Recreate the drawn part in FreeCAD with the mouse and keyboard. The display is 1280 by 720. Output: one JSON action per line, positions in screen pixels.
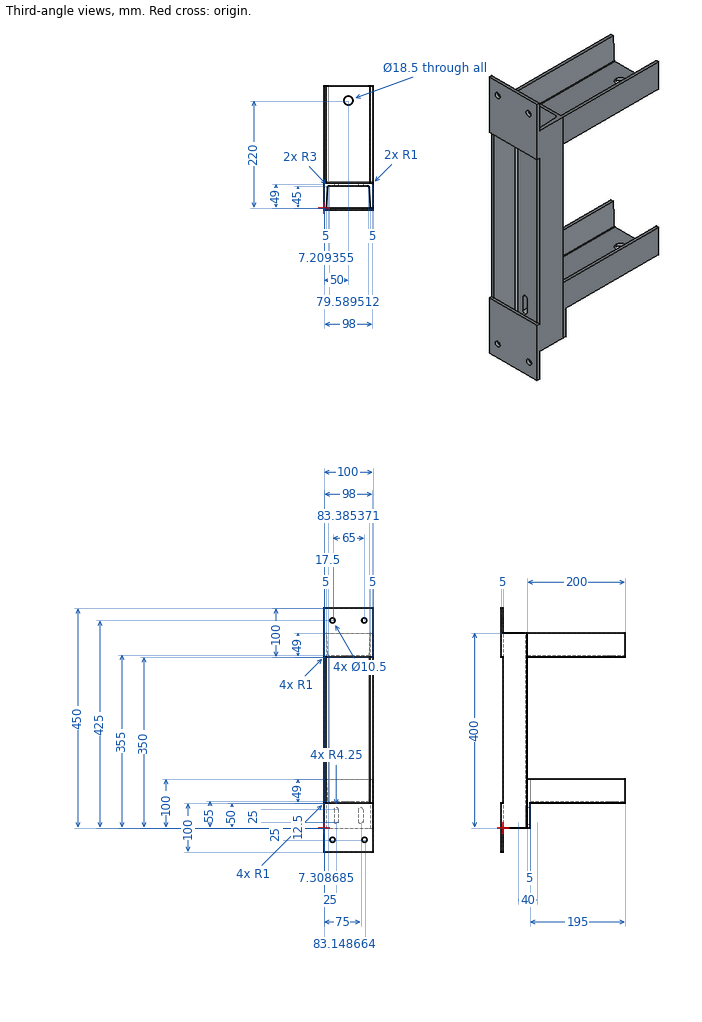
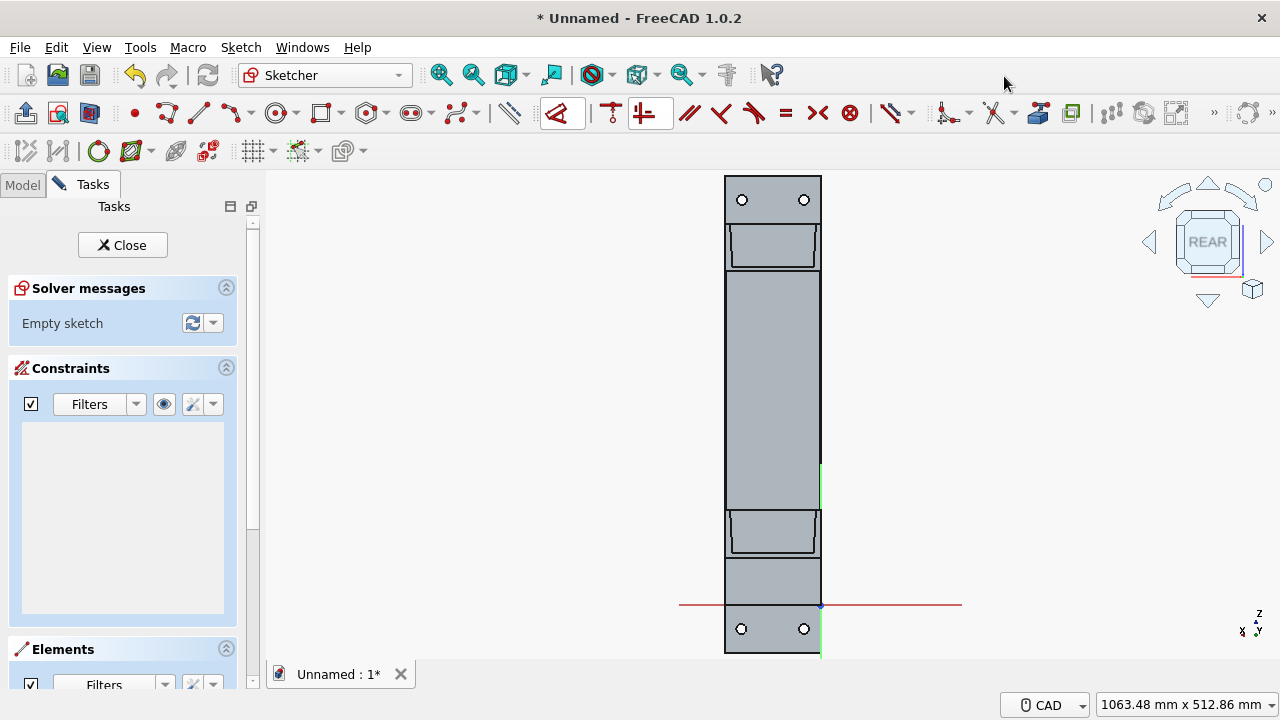
{"action": "left_click", "coordinate": [90, 114]}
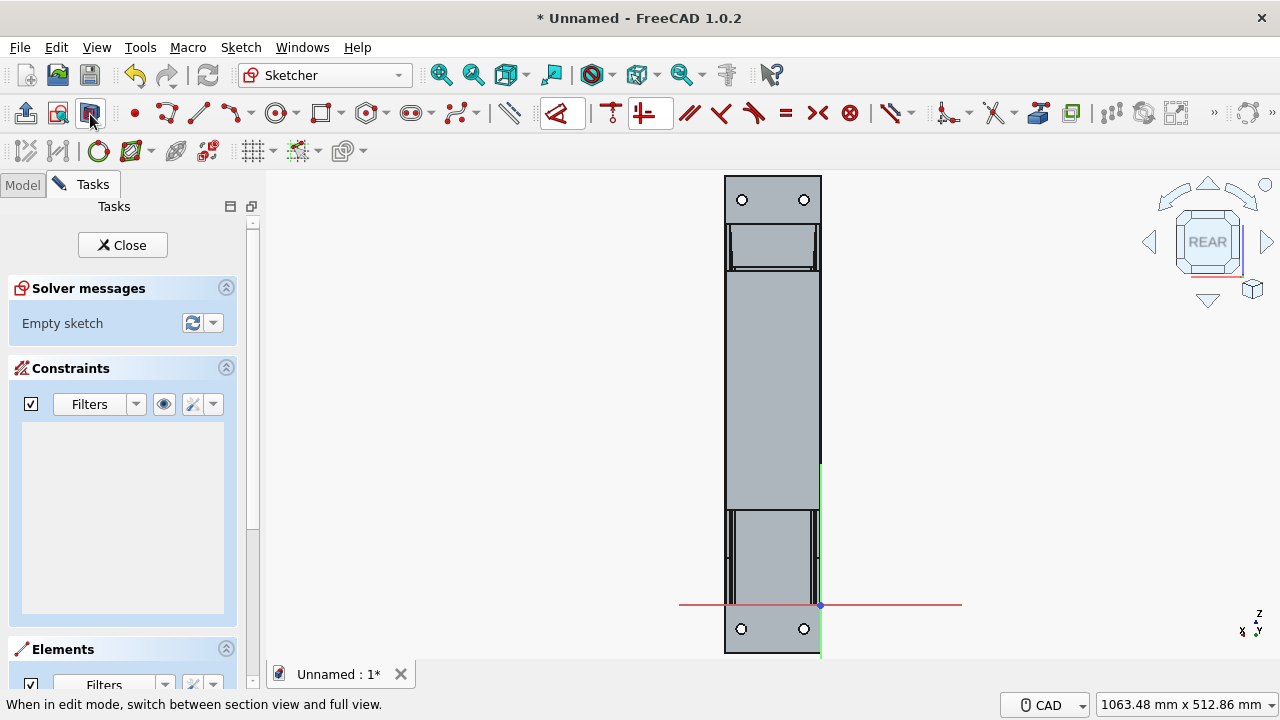
{"action": "scroll", "coordinate": [795, 612], "scroll_direction": "up", "scroll_amount": 10}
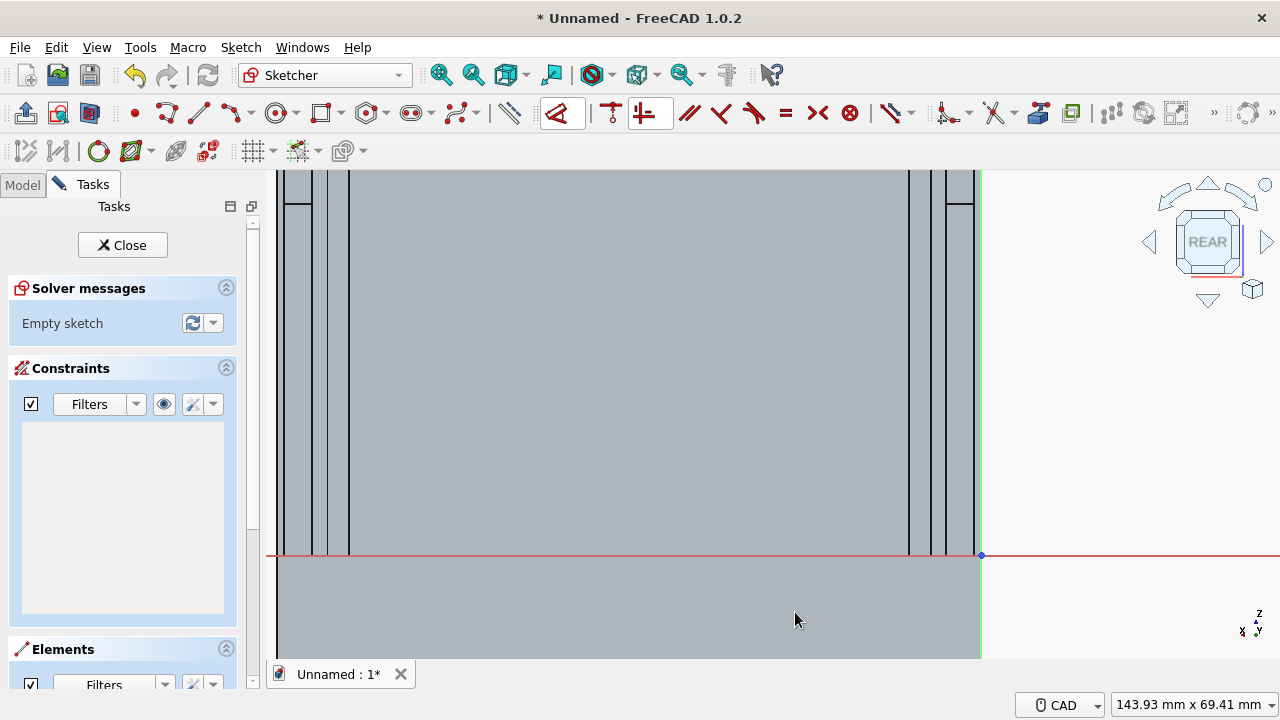
{"action": "left_click", "coordinate": [412, 114]}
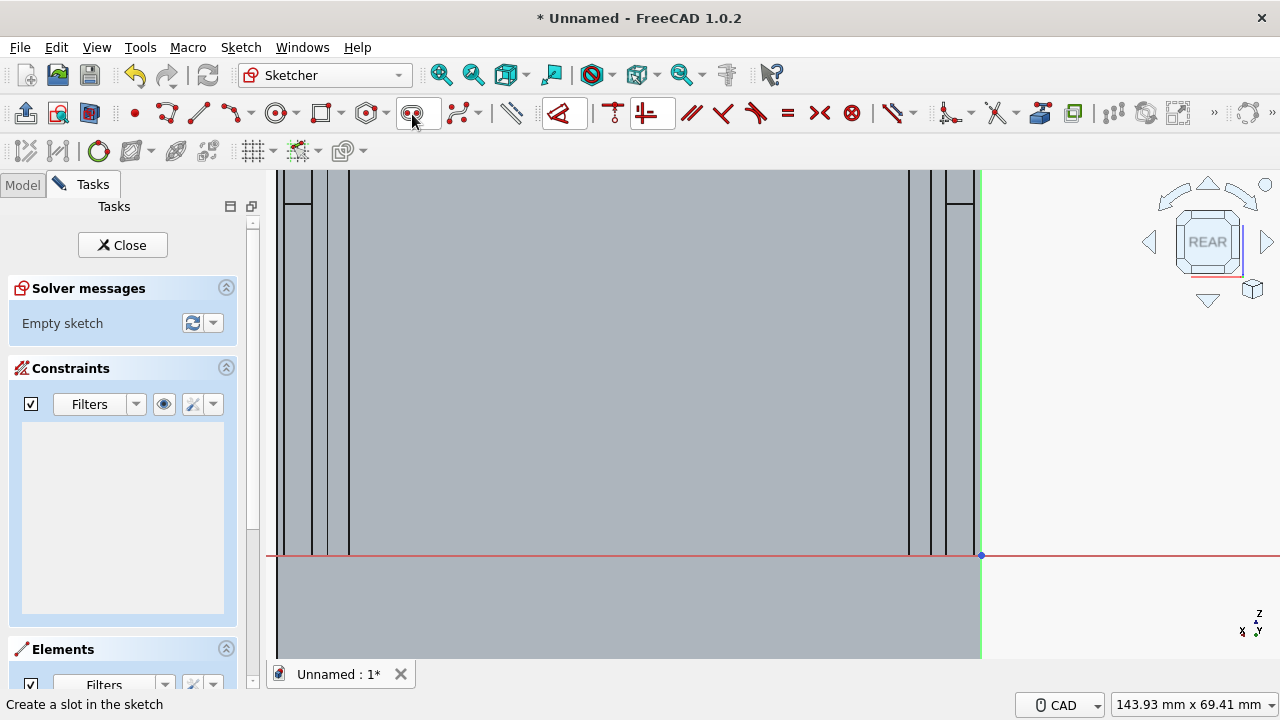
{"action": "left_click", "coordinate": [805, 468]}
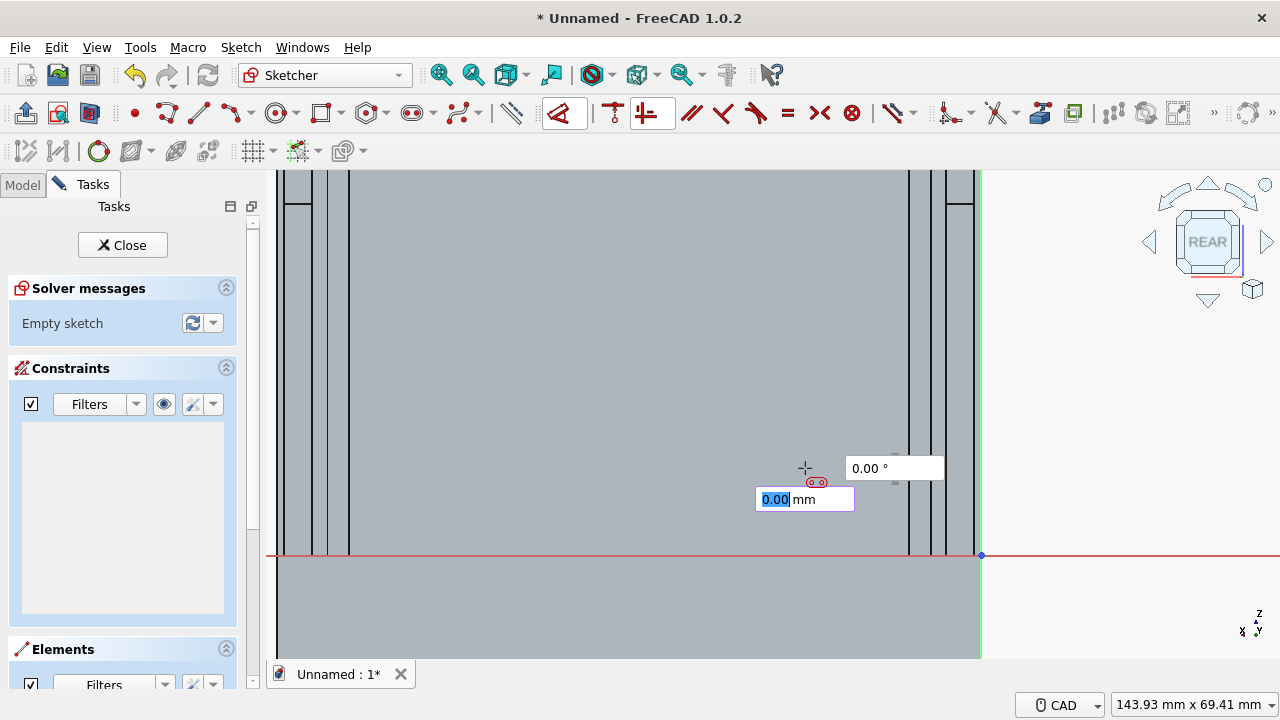
{"action": "left_click", "coordinate": [805, 292]}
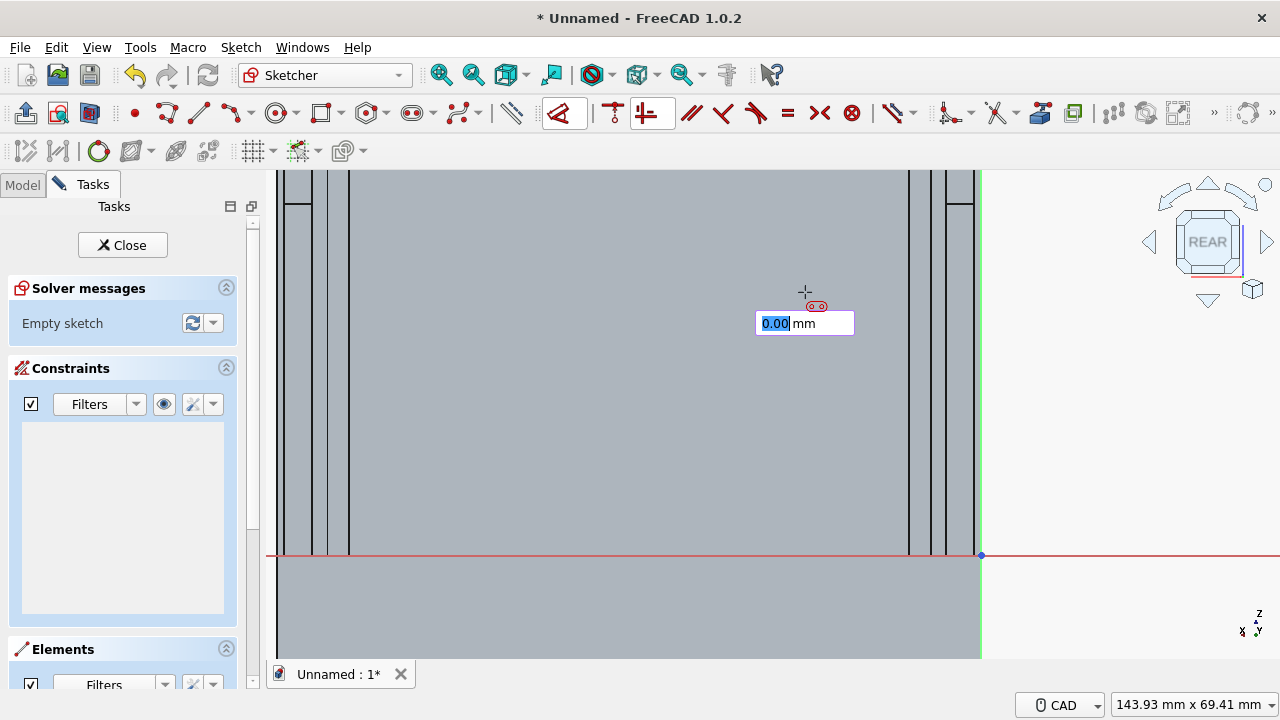
{"action": "left_click", "coordinate": [835, 380]}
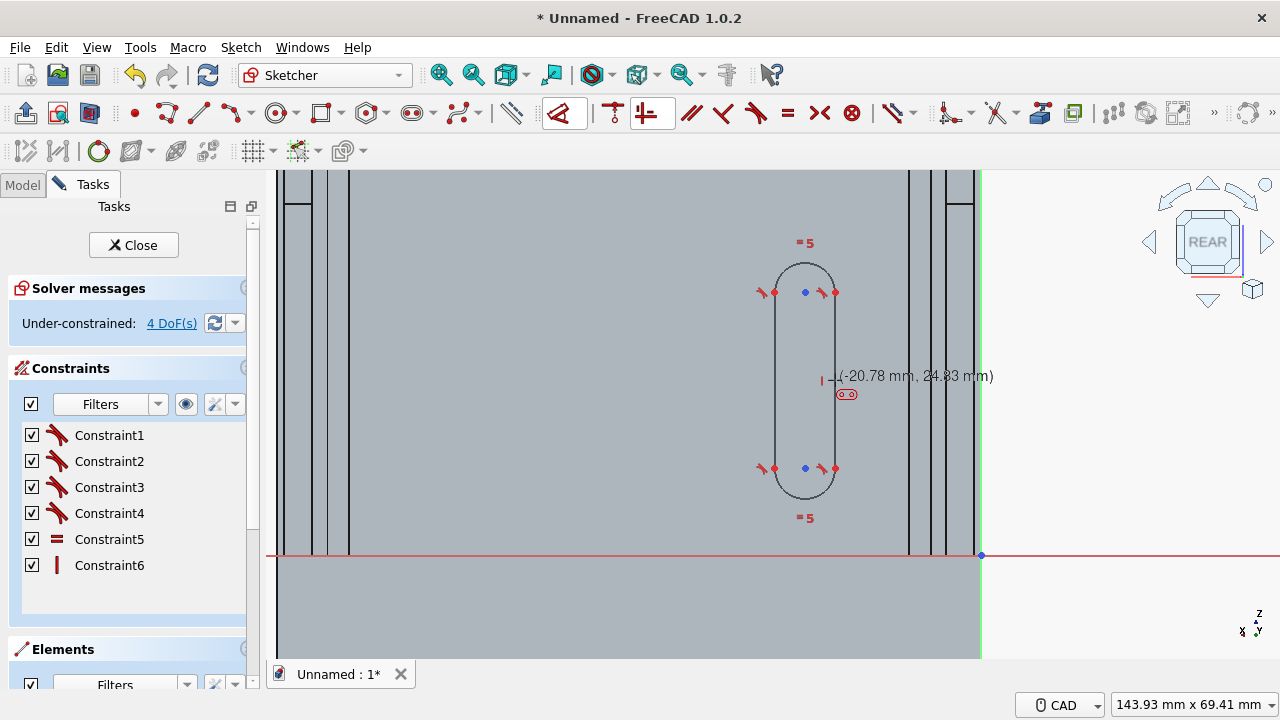
{"action": "left_click", "coordinate": [453, 468]}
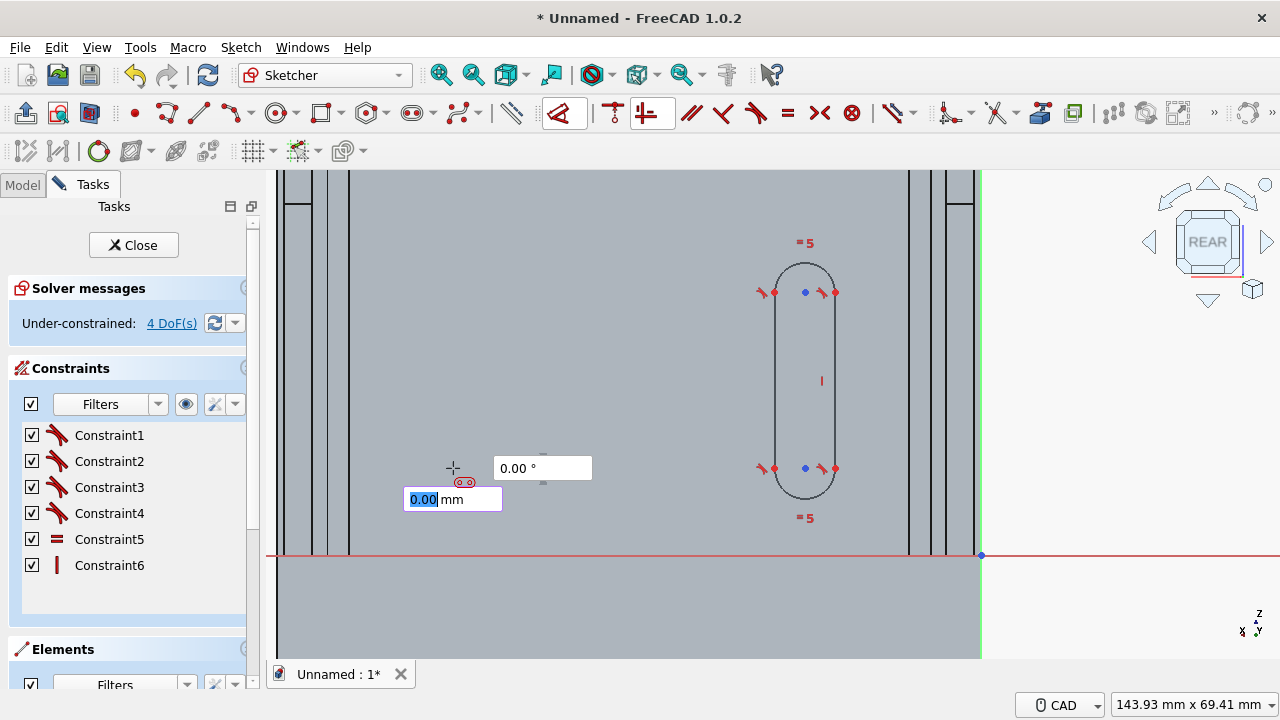
{"action": "left_click", "coordinate": [453, 292]}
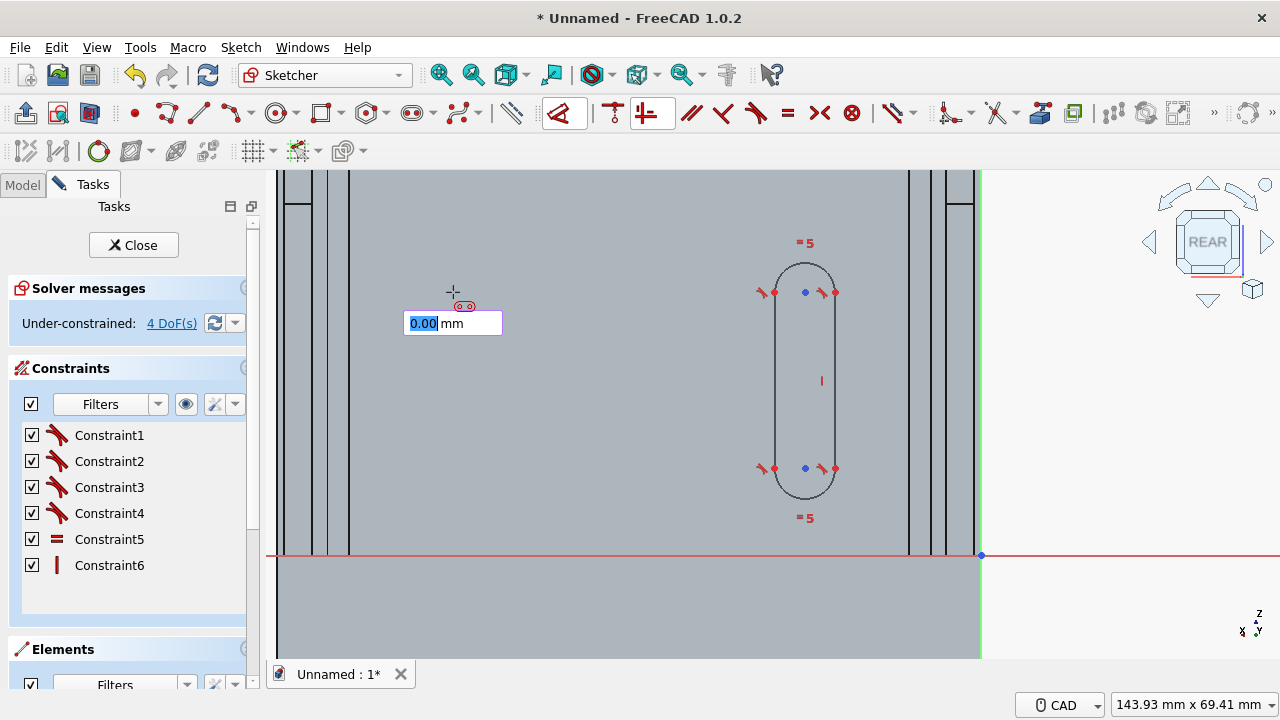
{"action": "left_click", "coordinate": [483, 380]}
{"action": "key", "text": "Escape"}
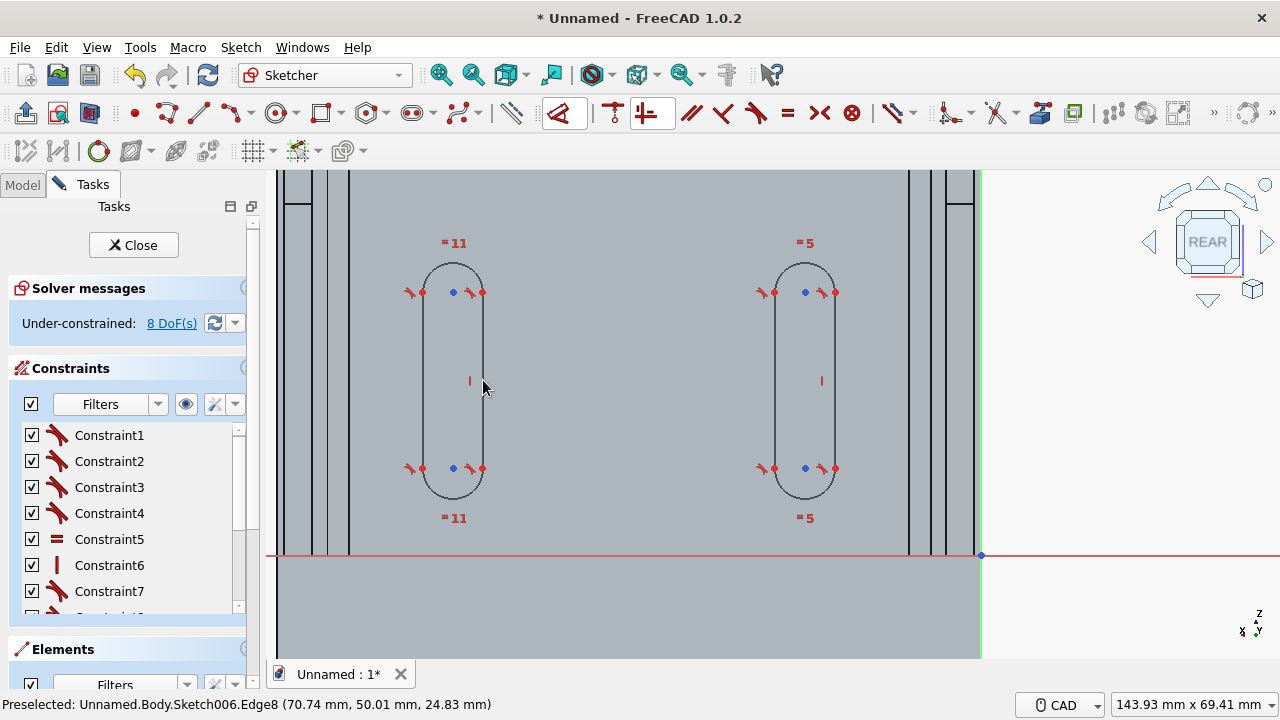
{"action": "left_click", "coordinate": [787, 493]}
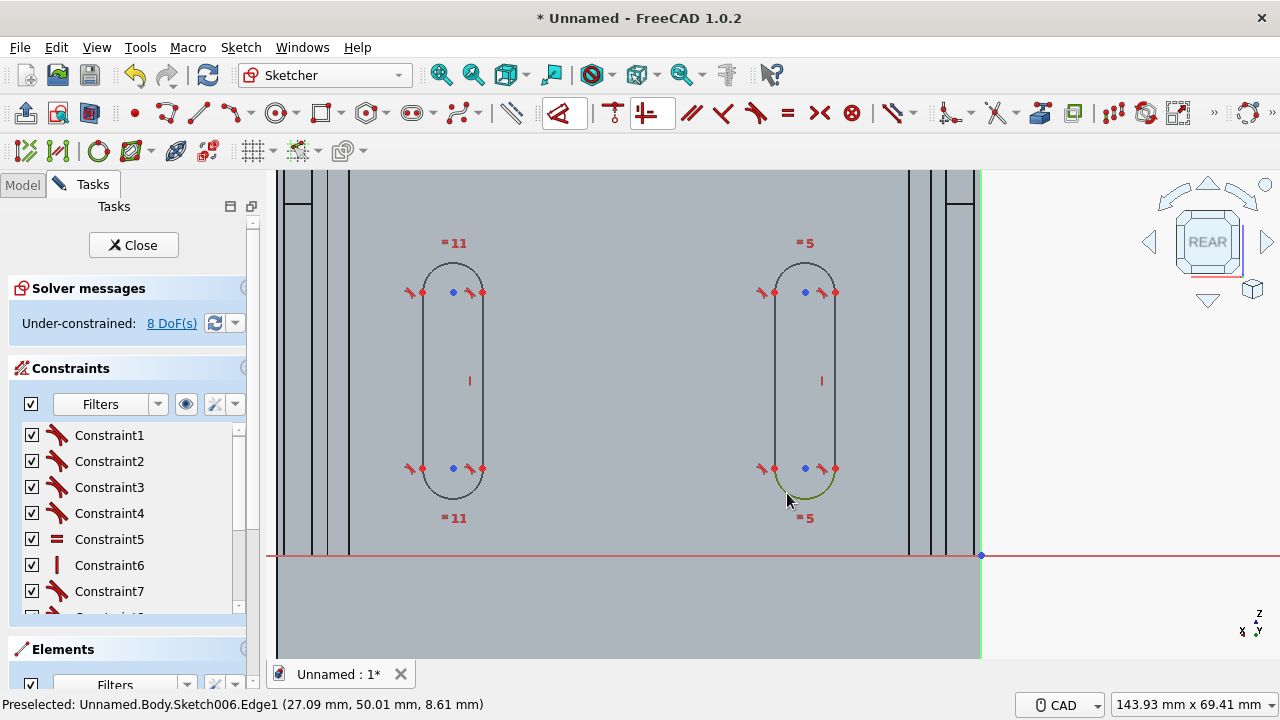
{"action": "left_click", "coordinate": [435, 493]}